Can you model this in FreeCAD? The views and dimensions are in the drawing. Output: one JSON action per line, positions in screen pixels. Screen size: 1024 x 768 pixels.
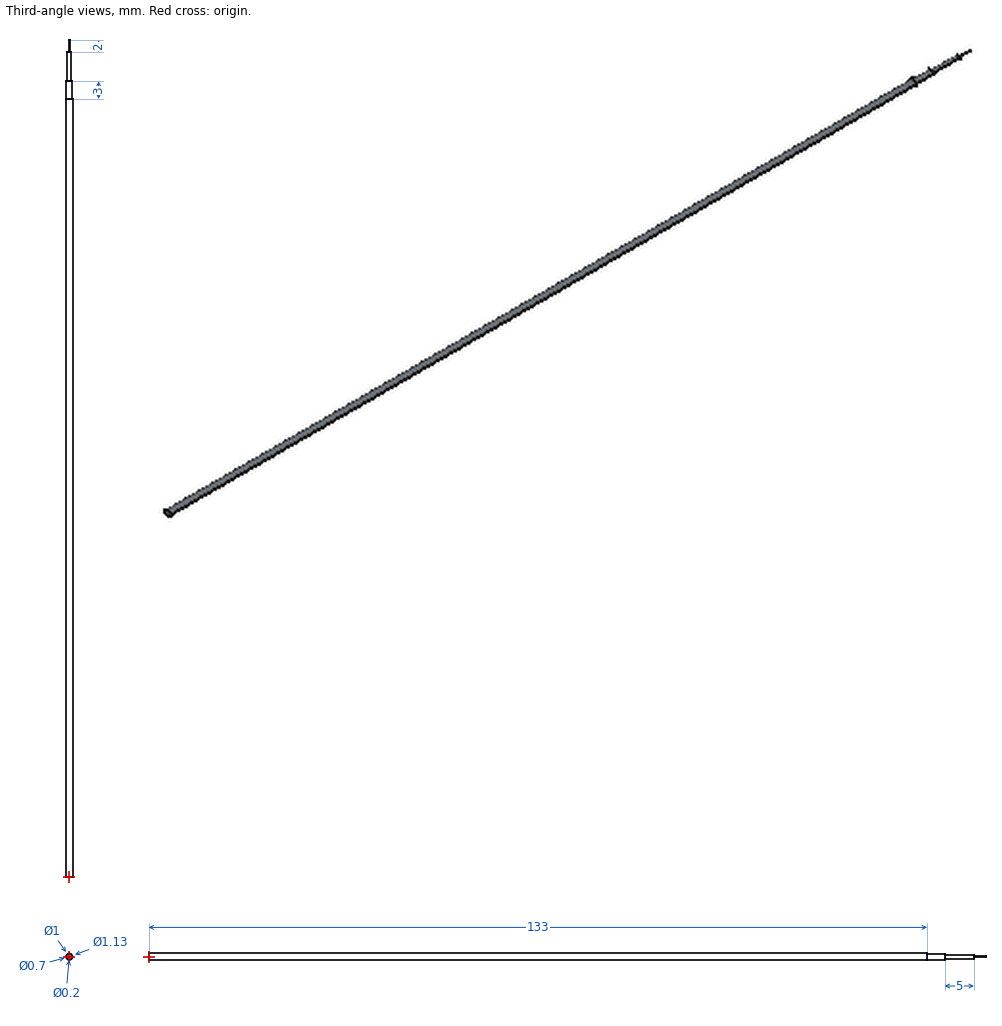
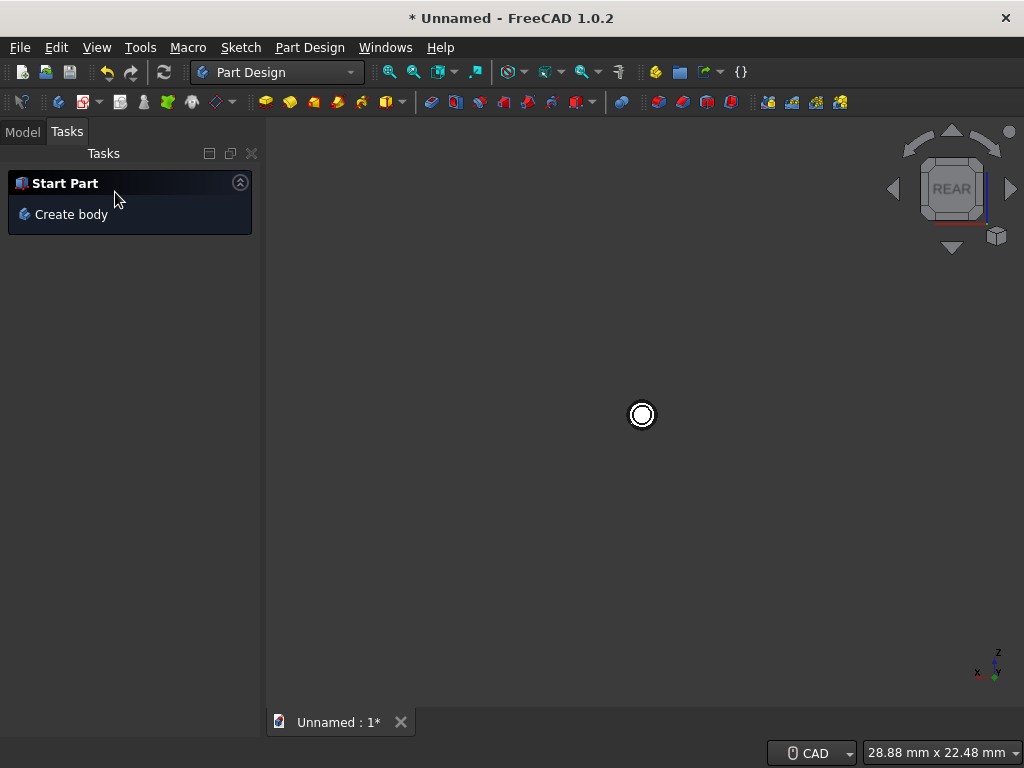
{"action": "left_click", "coordinate": [390, 72]}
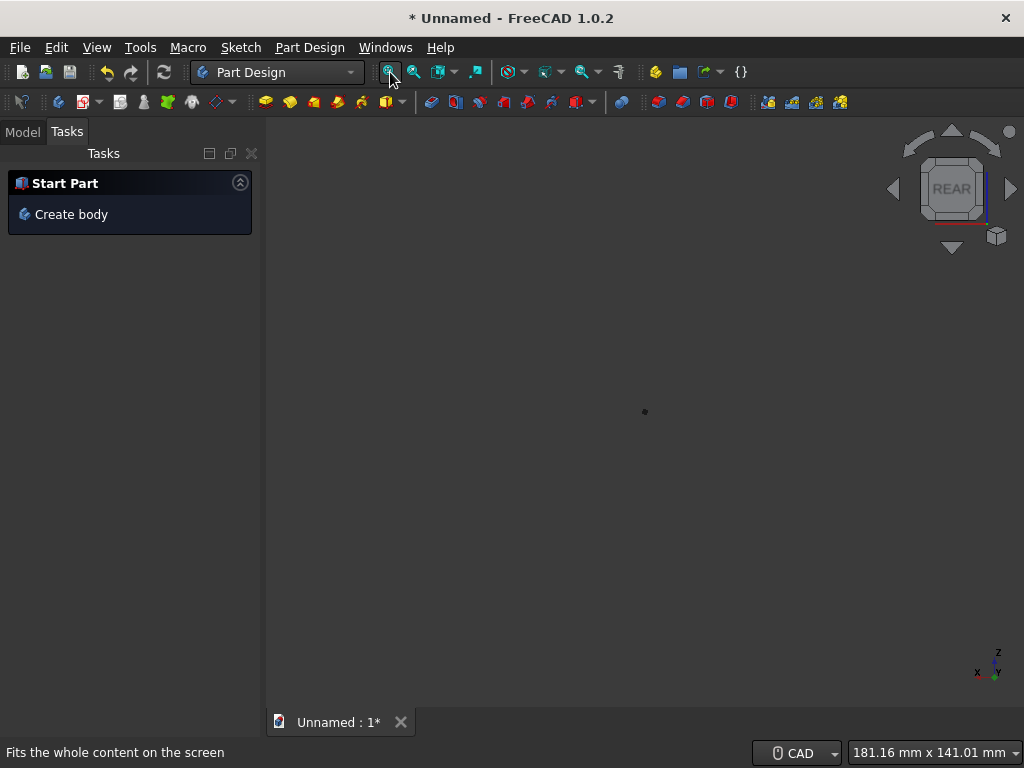
{"action": "scroll", "coordinate": [645, 411], "scroll_direction": "up", "scroll_amount": 11}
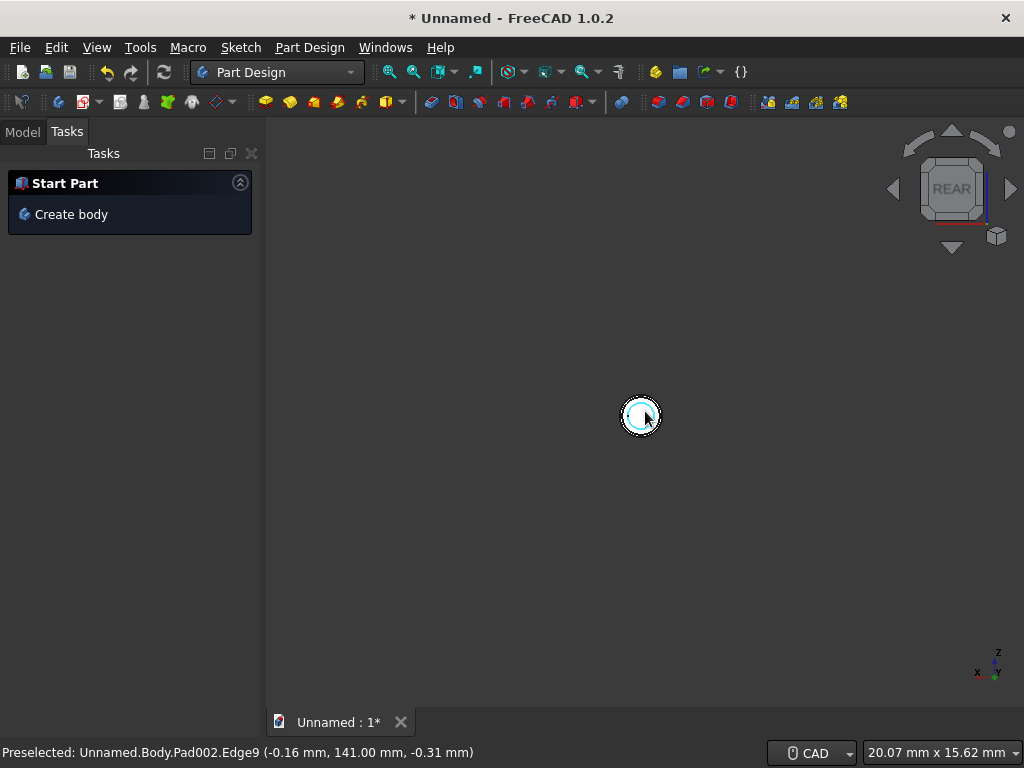
{"action": "left_click", "coordinate": [641, 415]}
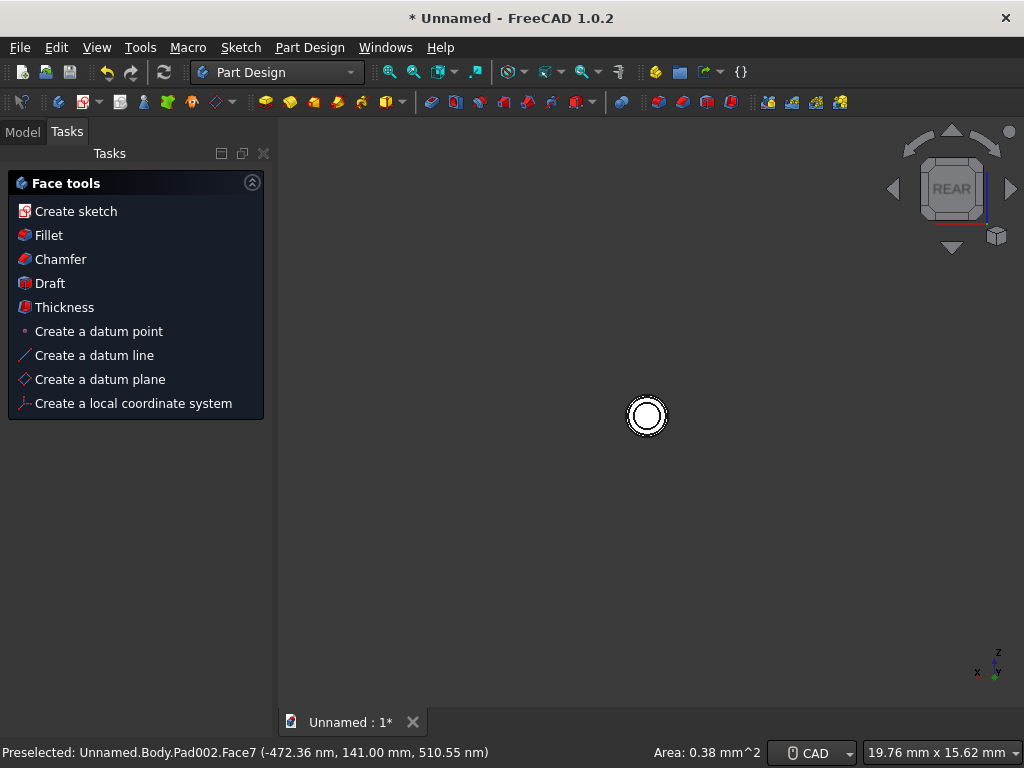
{"action": "left_click", "coordinate": [84, 102]}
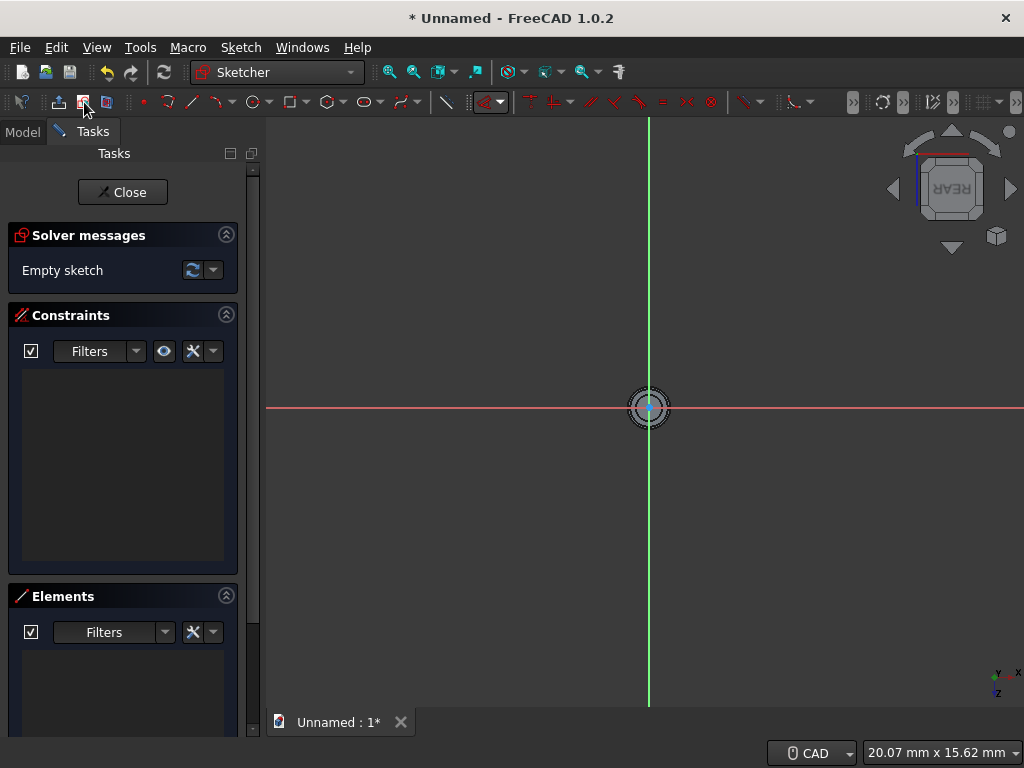
{"action": "scroll", "coordinate": [653, 408], "scroll_direction": "up", "scroll_amount": 15}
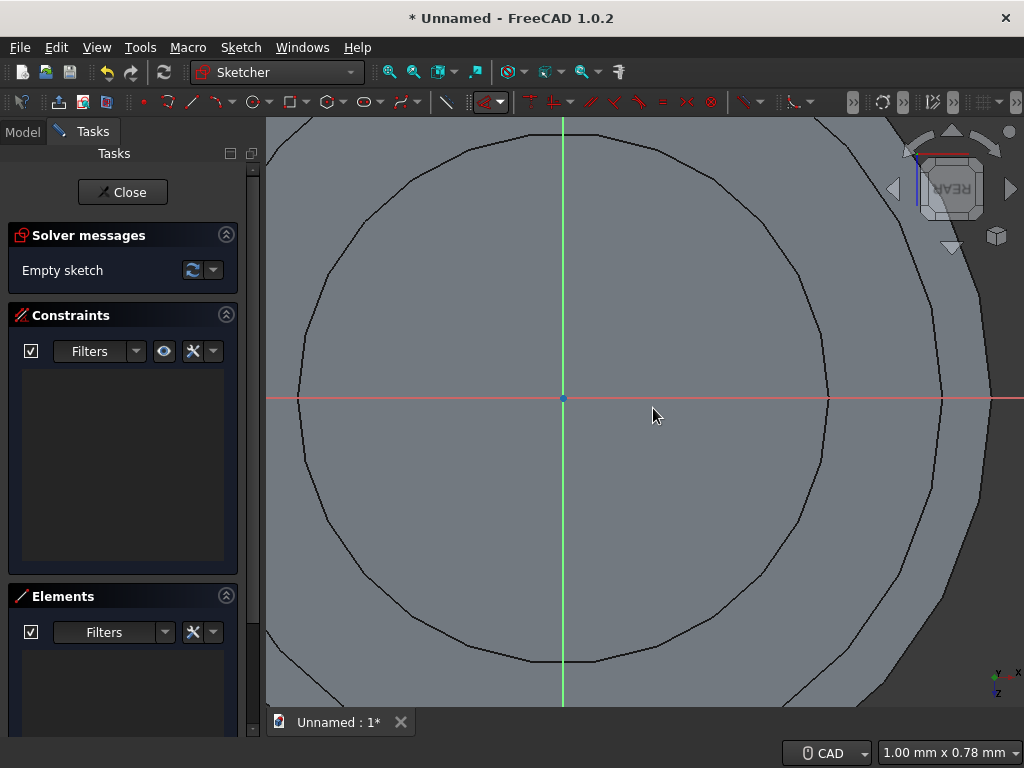
{"action": "scroll", "coordinate": [556, 390], "scroll_direction": "up", "scroll_amount": 5}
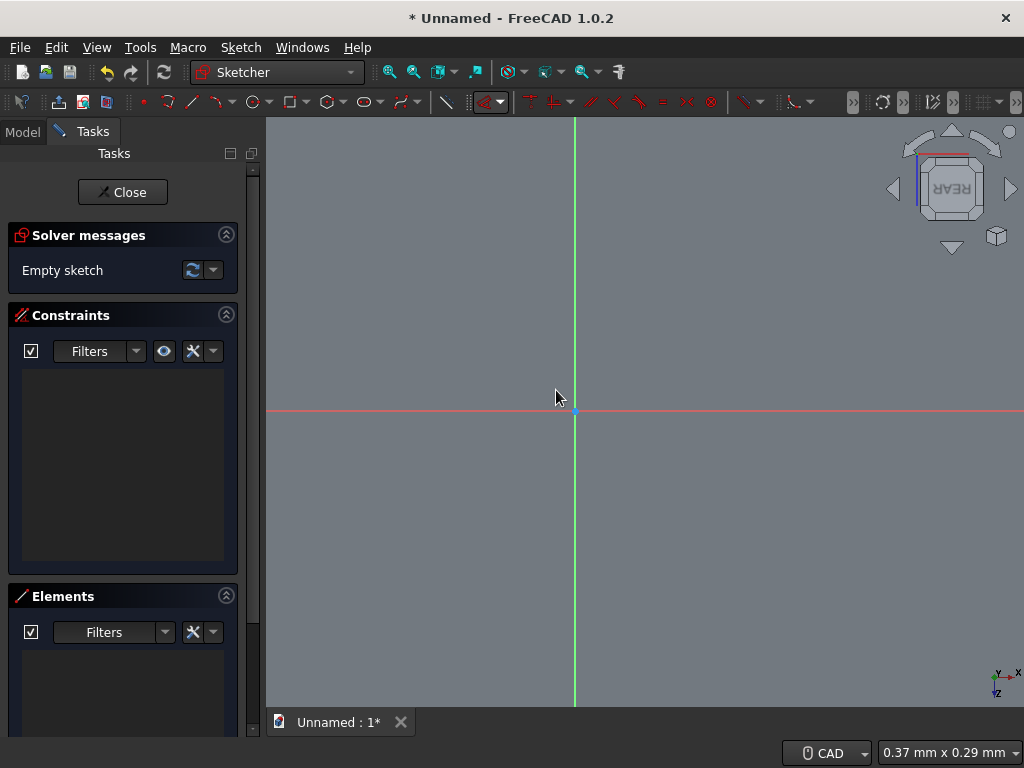
{"action": "key", "text": "g c"}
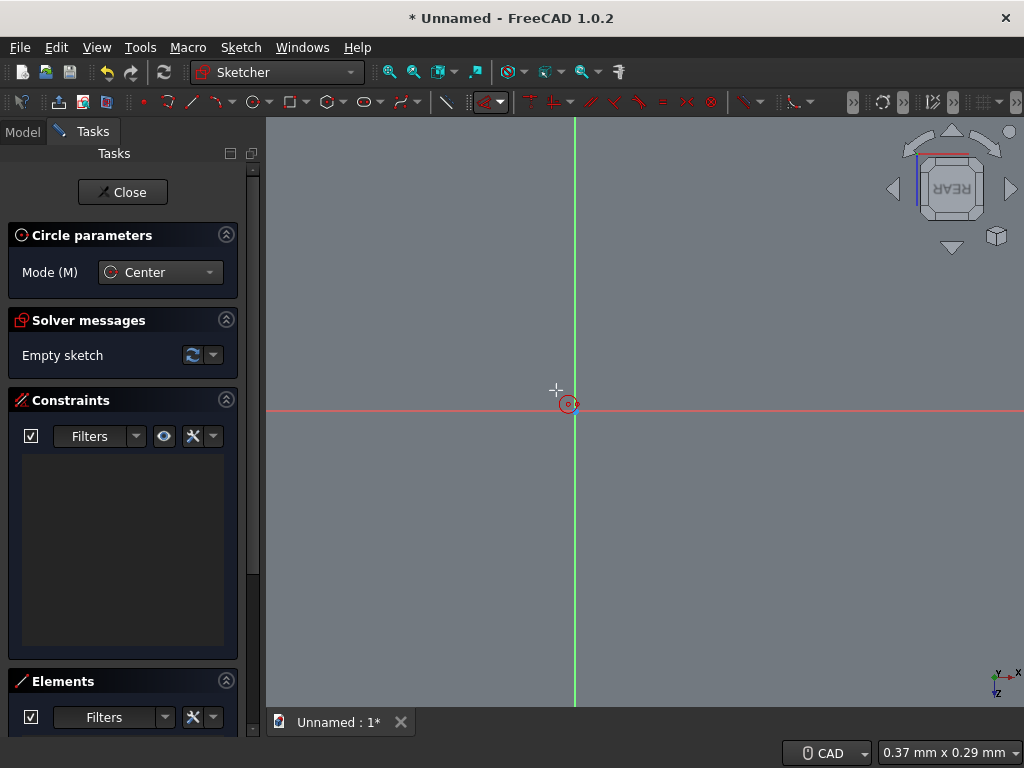
{"action": "left_click", "coordinate": [575, 411]}
{"action": "left_click", "coordinate": [721, 266]}
{"action": "key", "text": "Escape"}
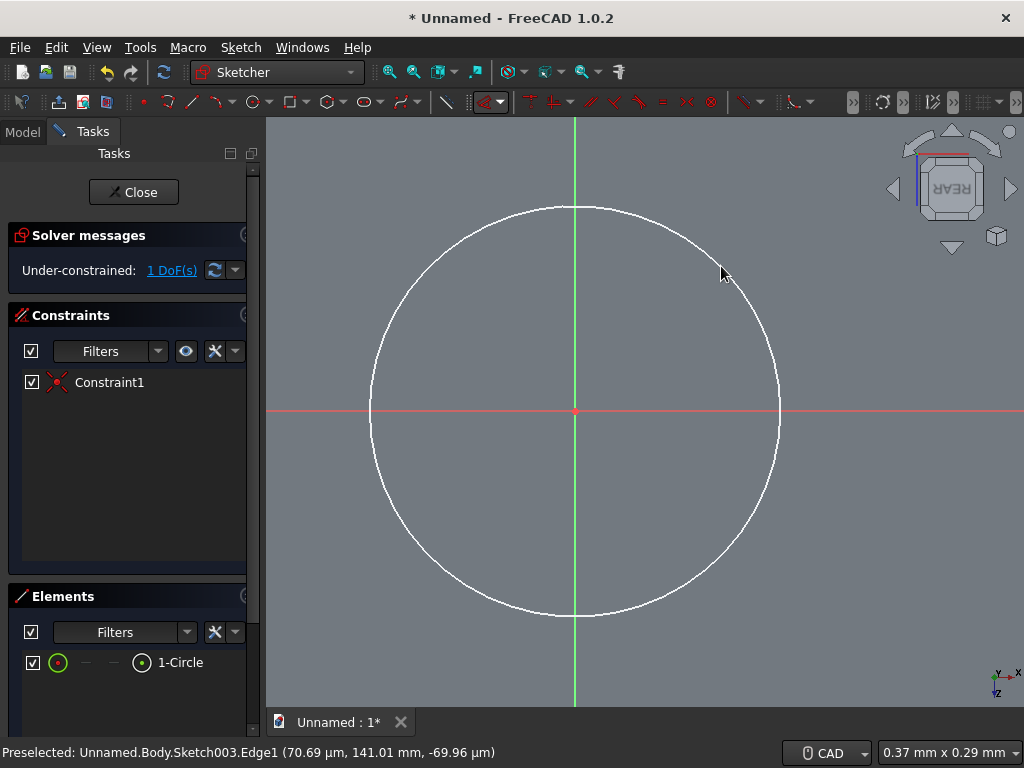
{"action": "left_click", "coordinate": [720, 266]}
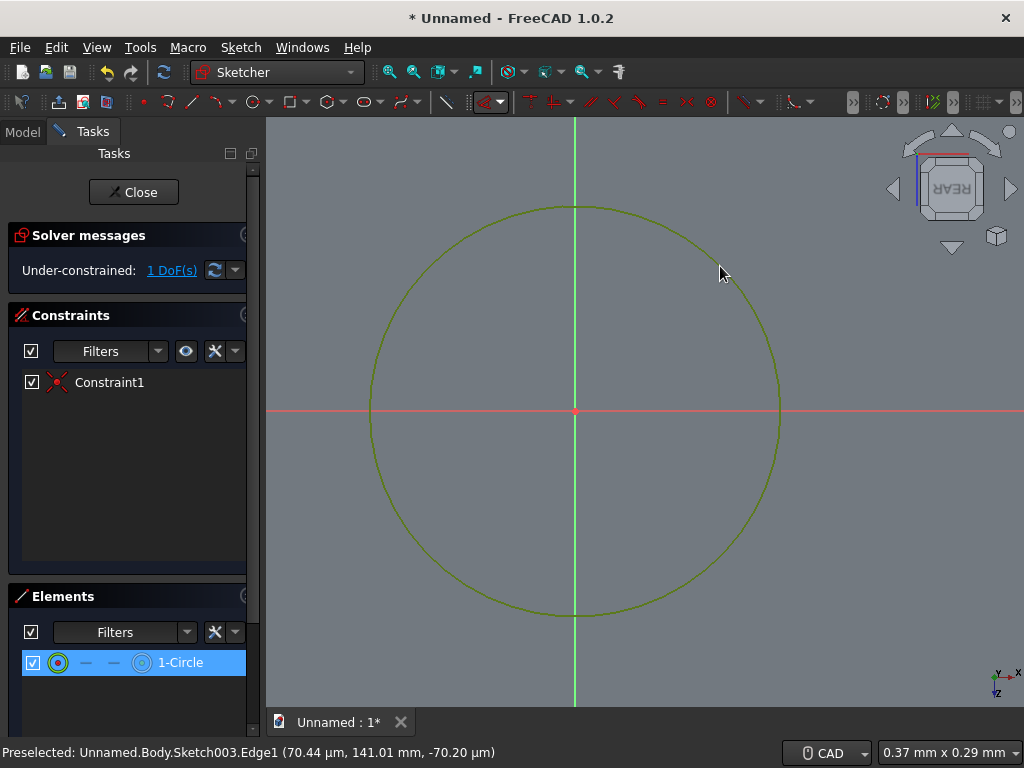
{"action": "key", "text": "k o"}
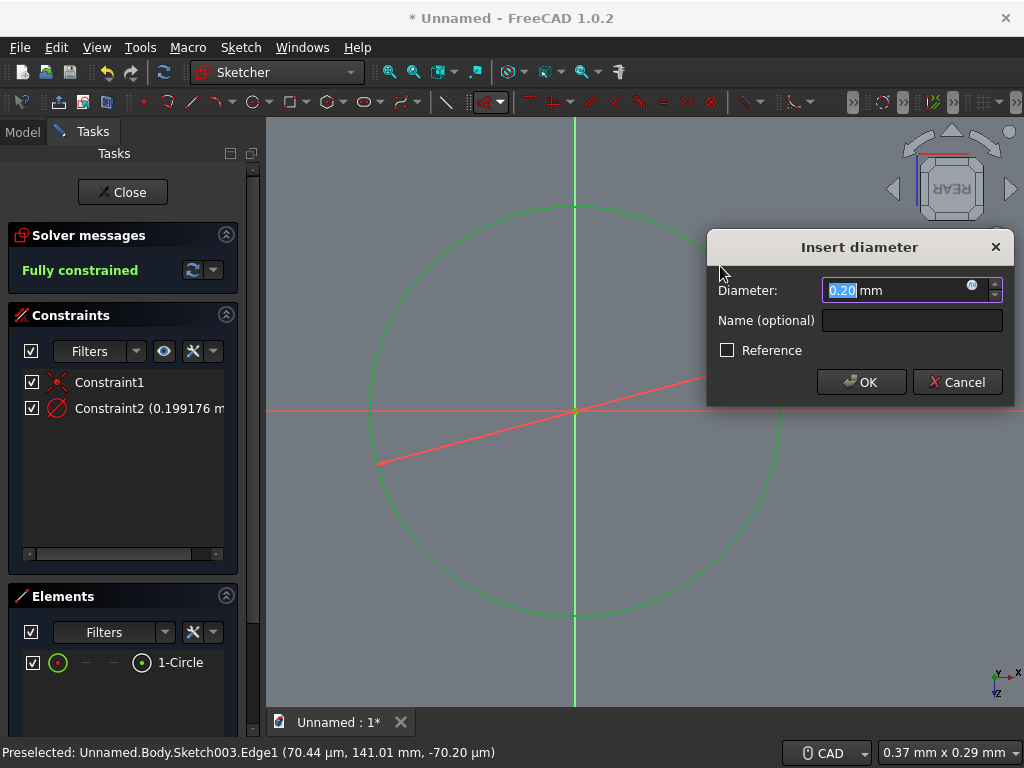
{"action": "type", "text": "0.2"}
{"action": "key", "text": "Return"}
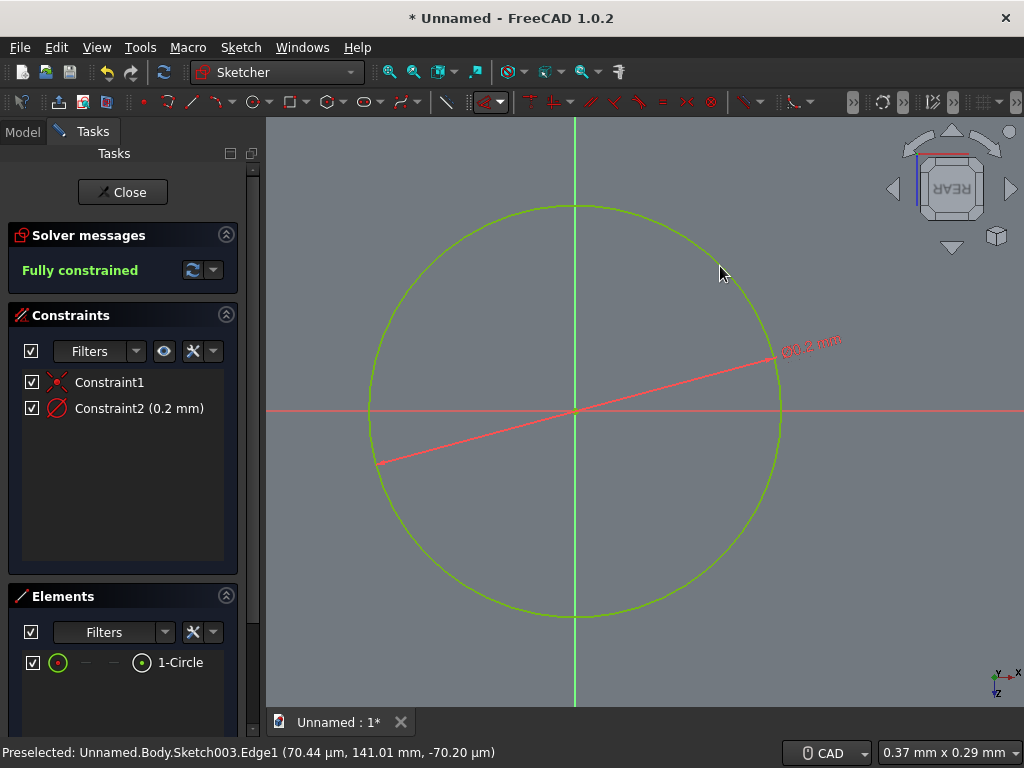
{"action": "left_click", "coordinate": [123, 192]}